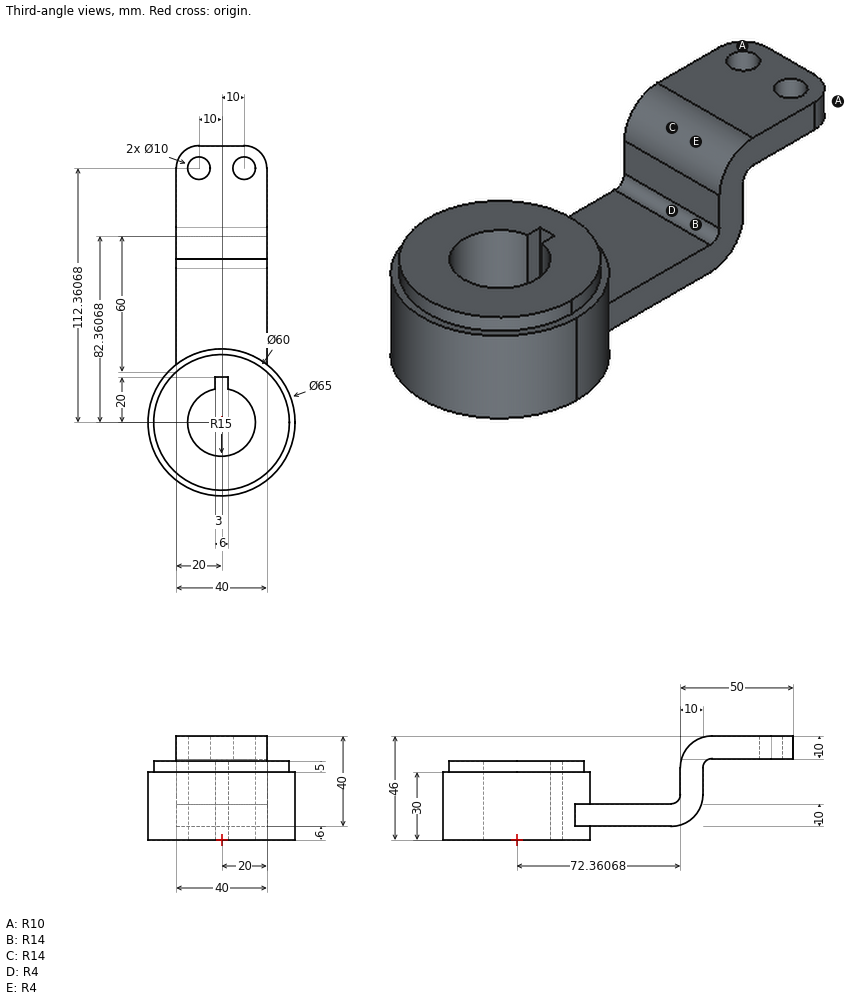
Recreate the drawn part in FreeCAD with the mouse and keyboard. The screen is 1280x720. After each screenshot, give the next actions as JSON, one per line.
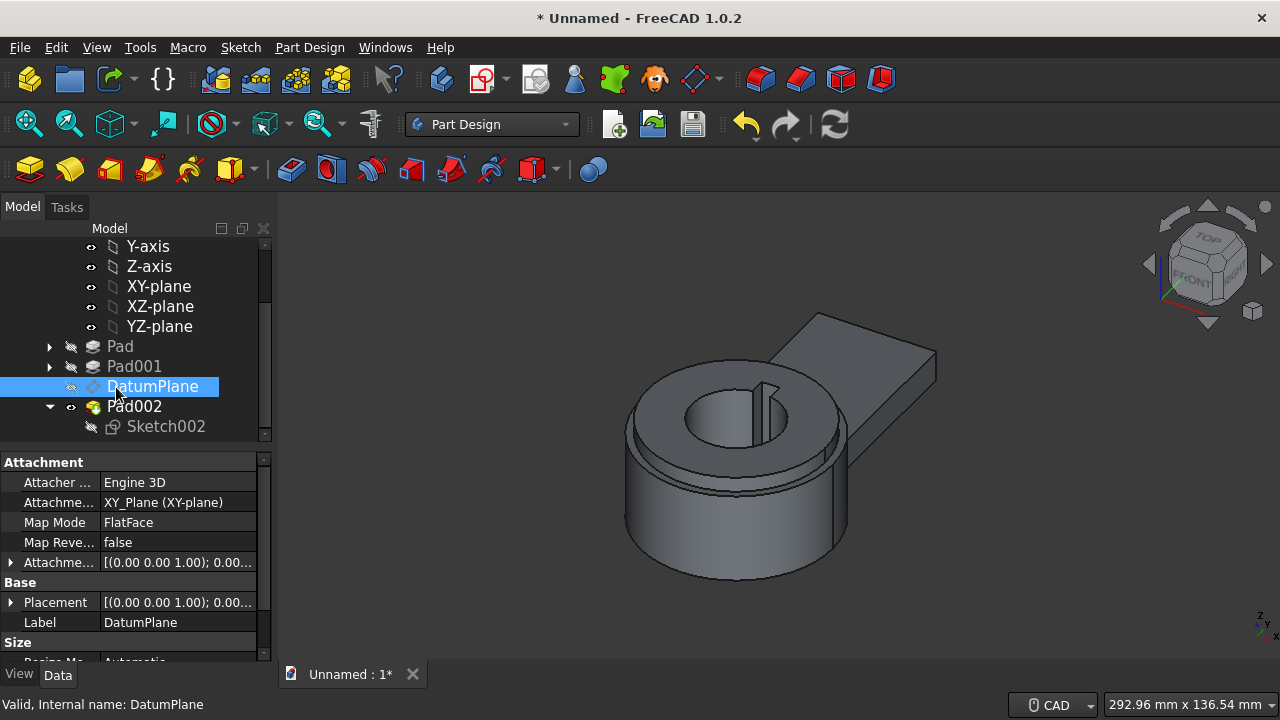
{"action": "key", "text": "4"}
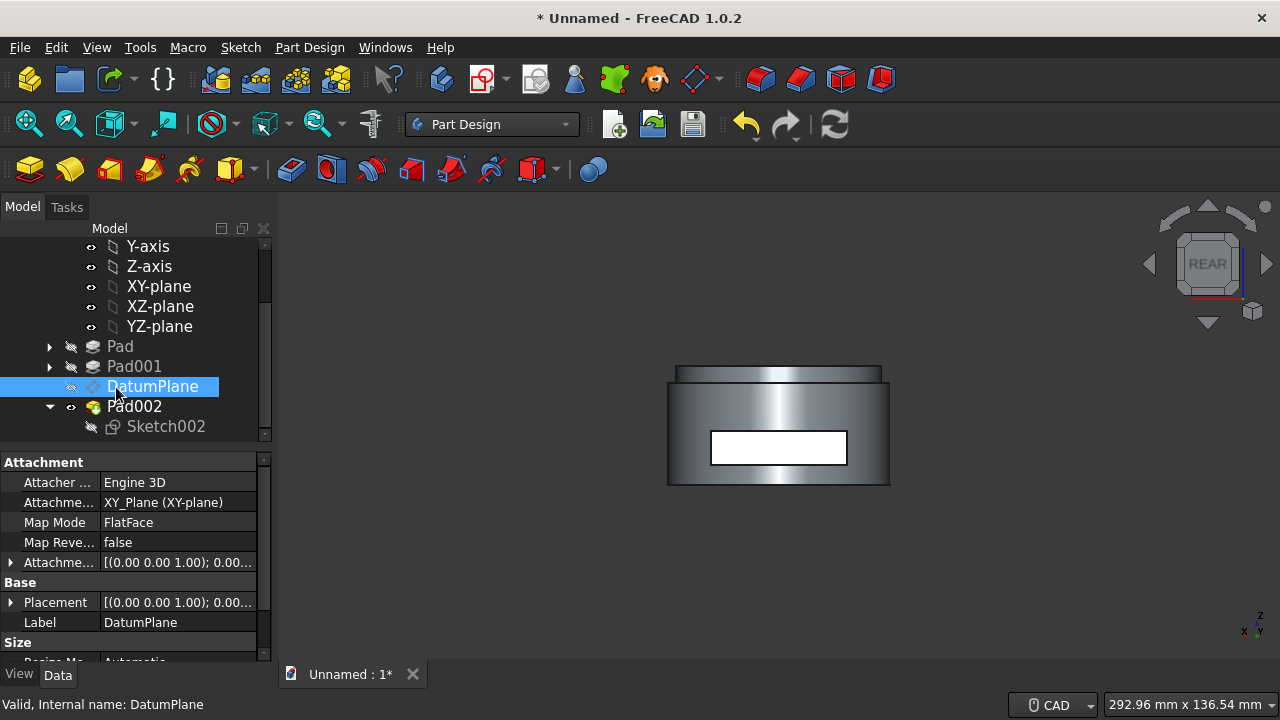
{"action": "key", "text": "v f"}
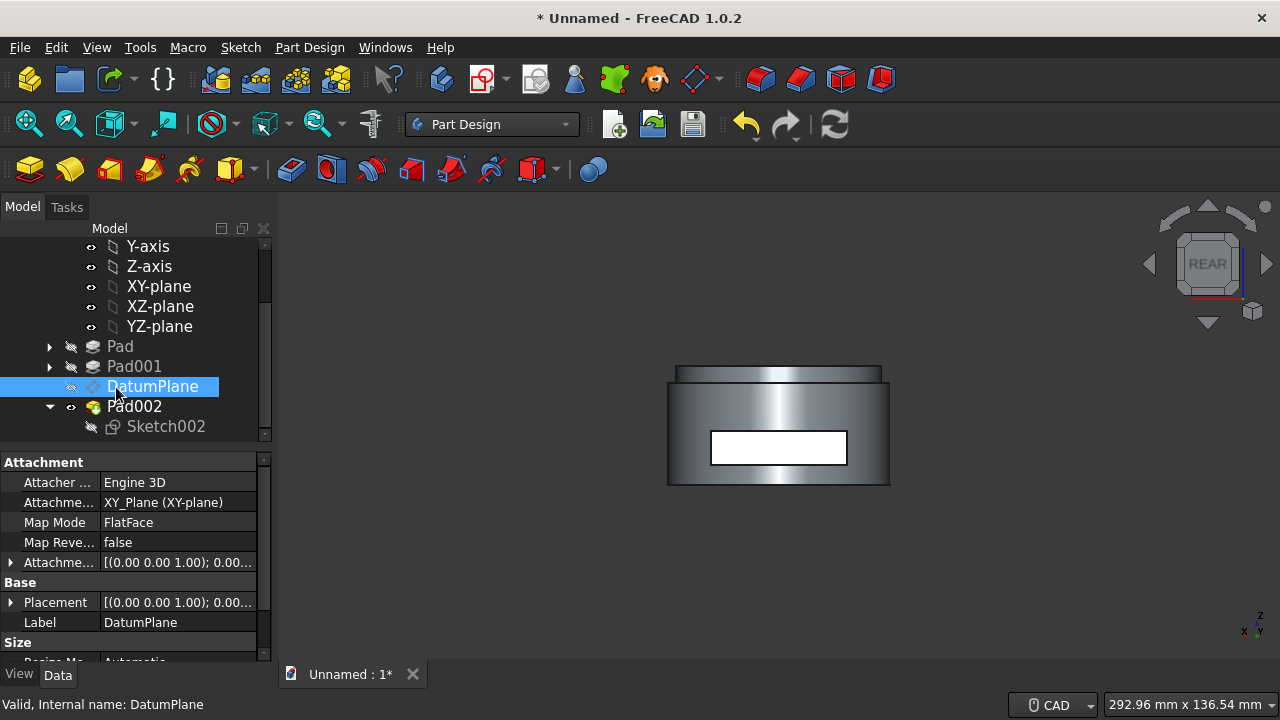
{"action": "left_click", "coordinate": [740, 447]}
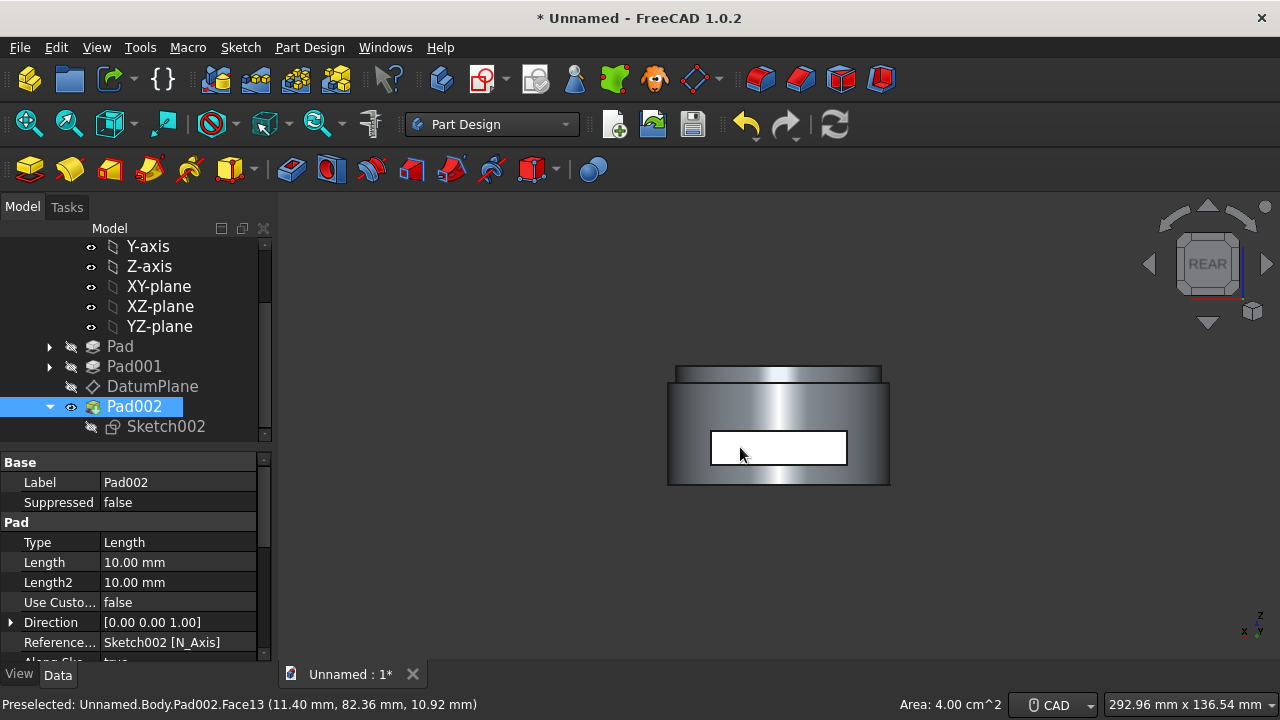
{"action": "left_click", "coordinate": [482, 80]}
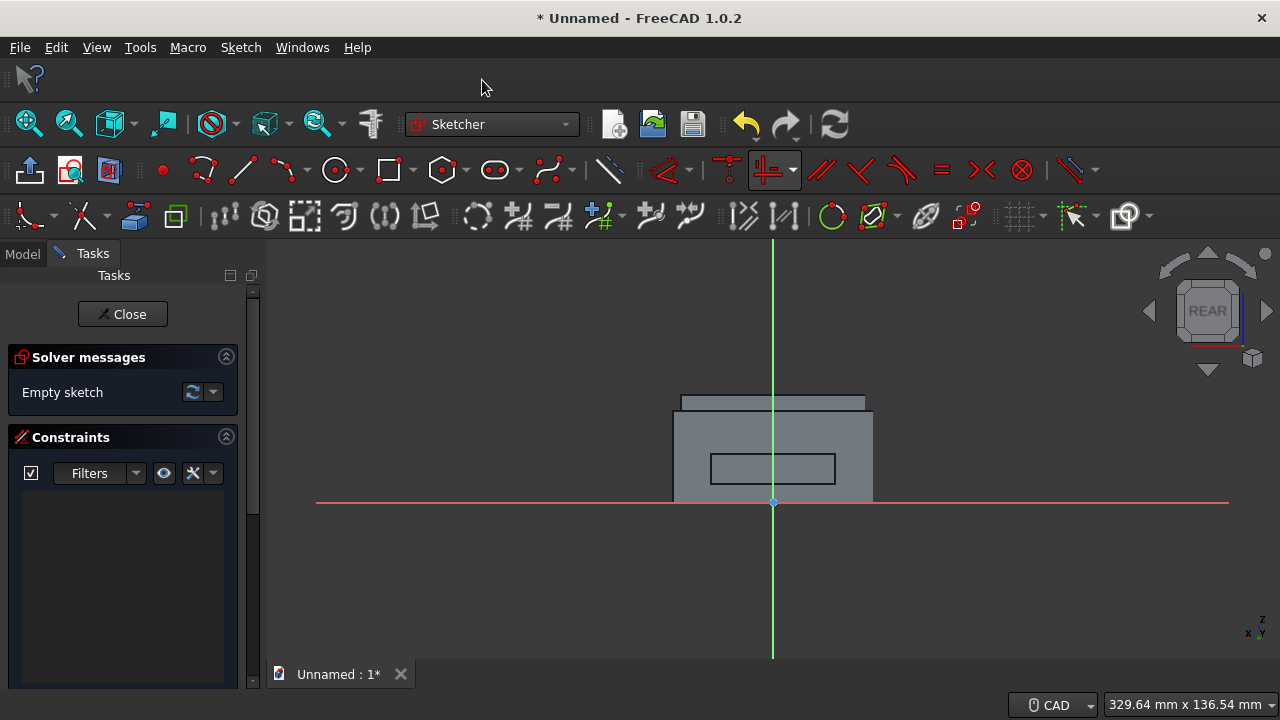
{"action": "scroll", "coordinate": [856, 412], "scroll_direction": "up", "scroll_amount": 3}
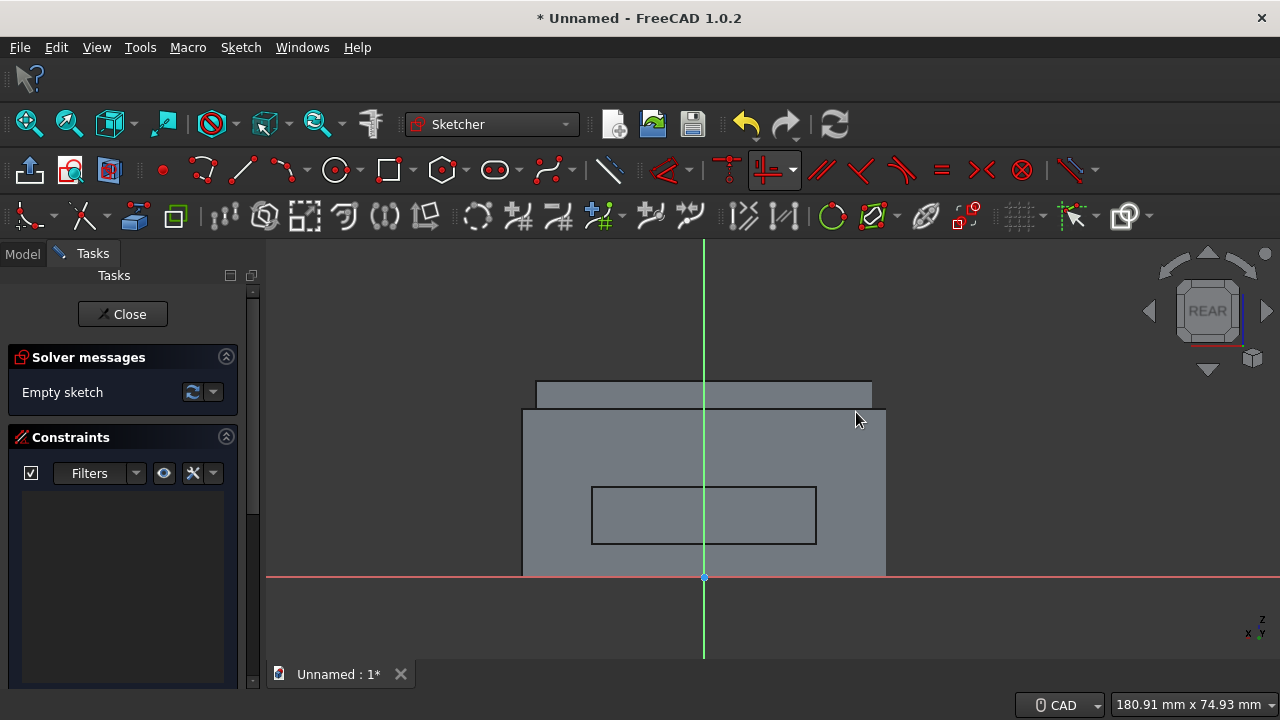
{"action": "key", "text": "g r"}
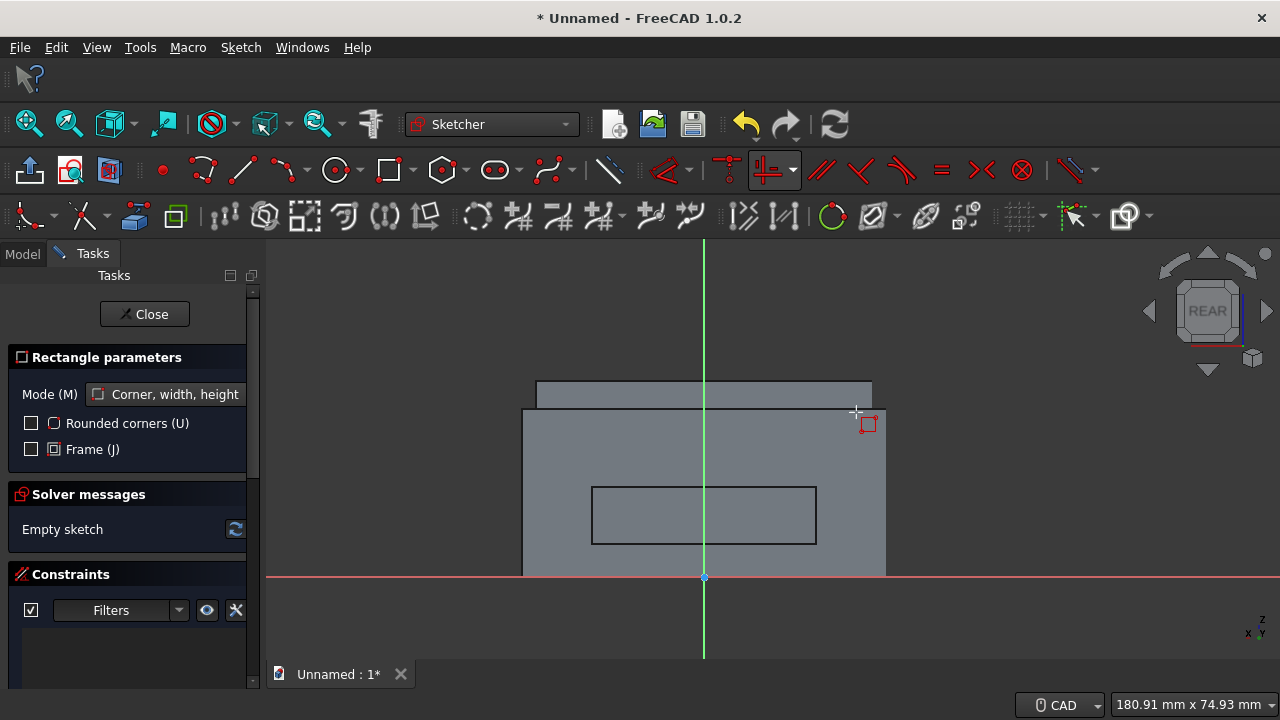
{"action": "left_click", "coordinate": [592, 319]}
{"action": "left_click", "coordinate": [816, 544]}
{"action": "key", "text": "Escape"}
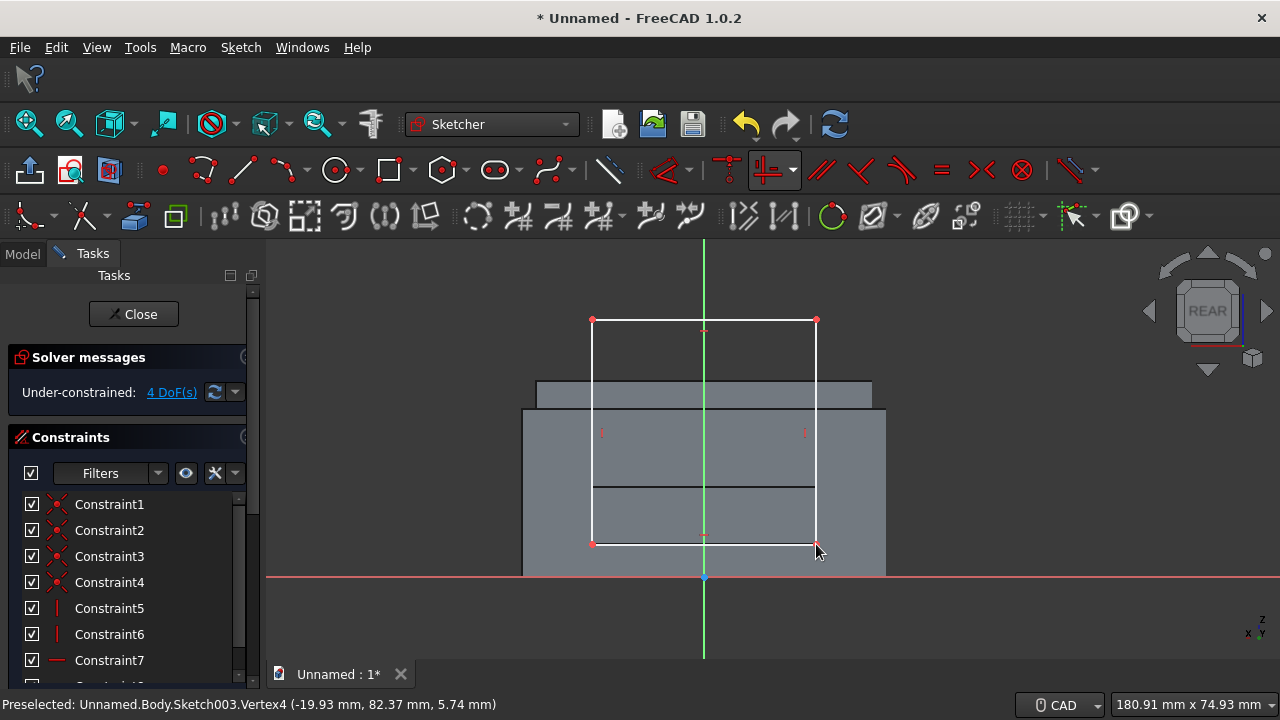
{"action": "key", "text": "d"}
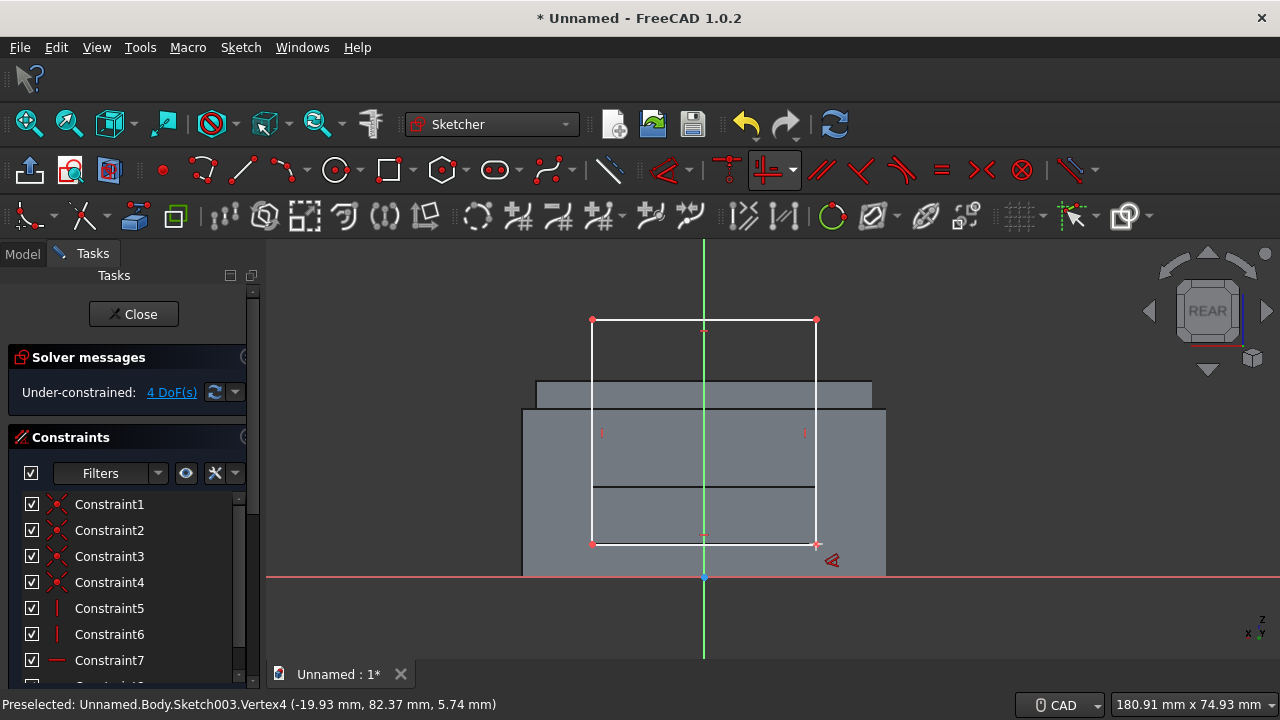
{"action": "left_click", "coordinate": [592, 387]}
{"action": "left_click", "coordinate": [558, 432]}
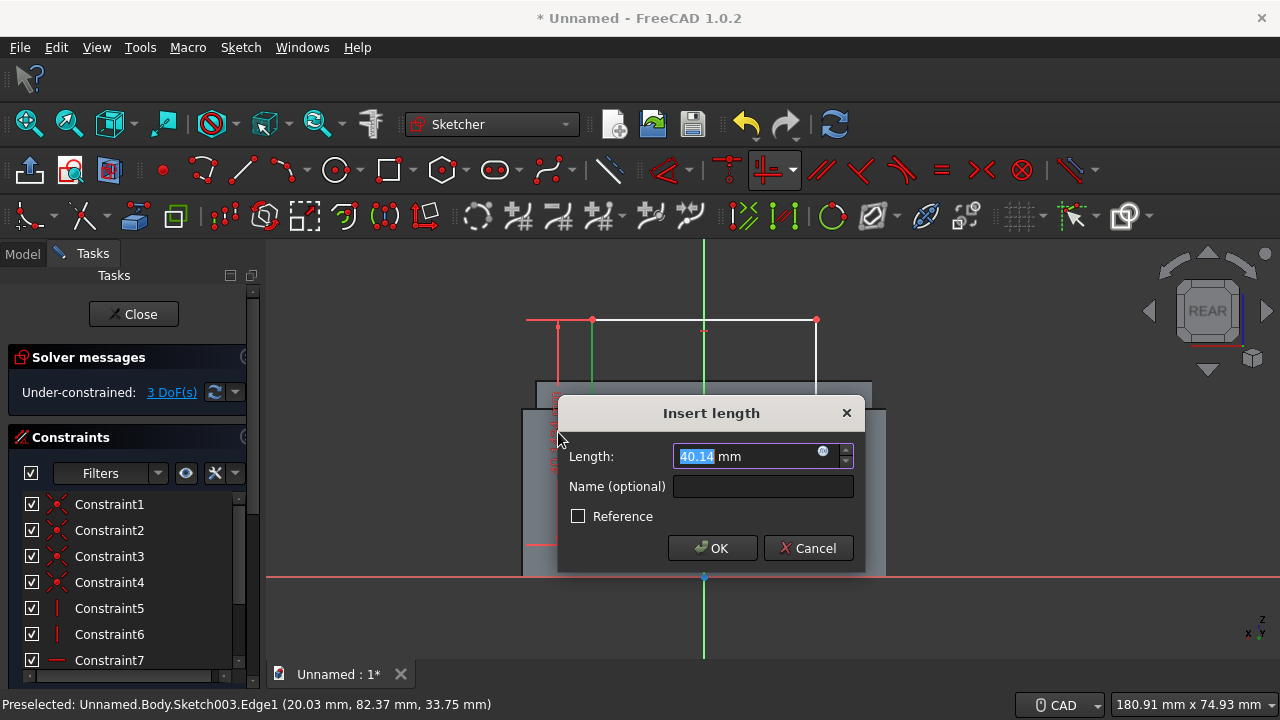
{"action": "type", "text": "40"}
{"action": "key", "text": "Return"}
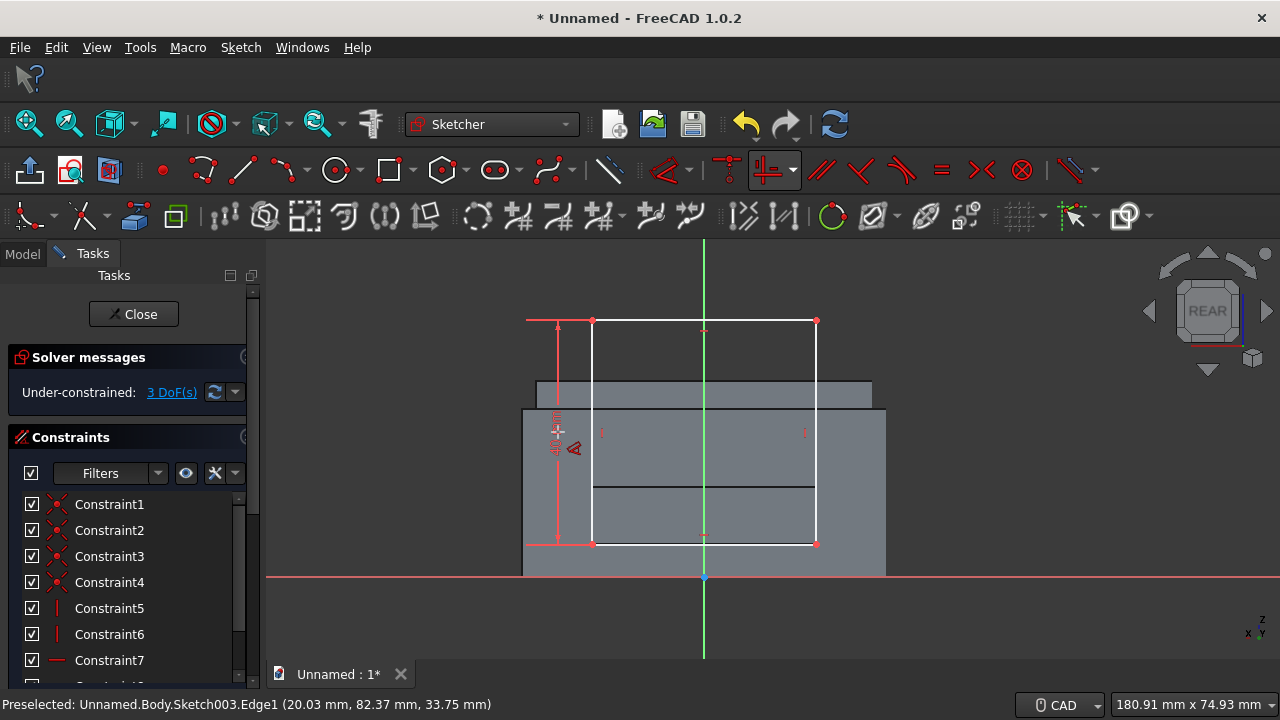
{"action": "left_click", "coordinate": [659, 545]}
{"action": "left_click", "coordinate": [652, 511]}